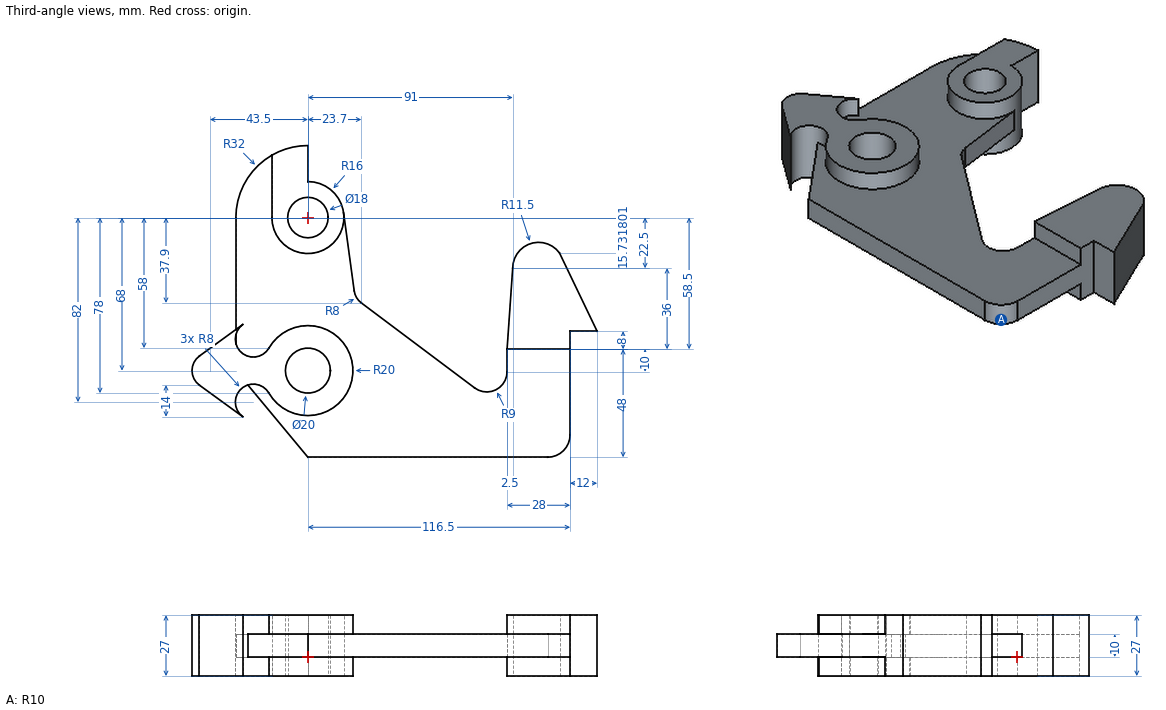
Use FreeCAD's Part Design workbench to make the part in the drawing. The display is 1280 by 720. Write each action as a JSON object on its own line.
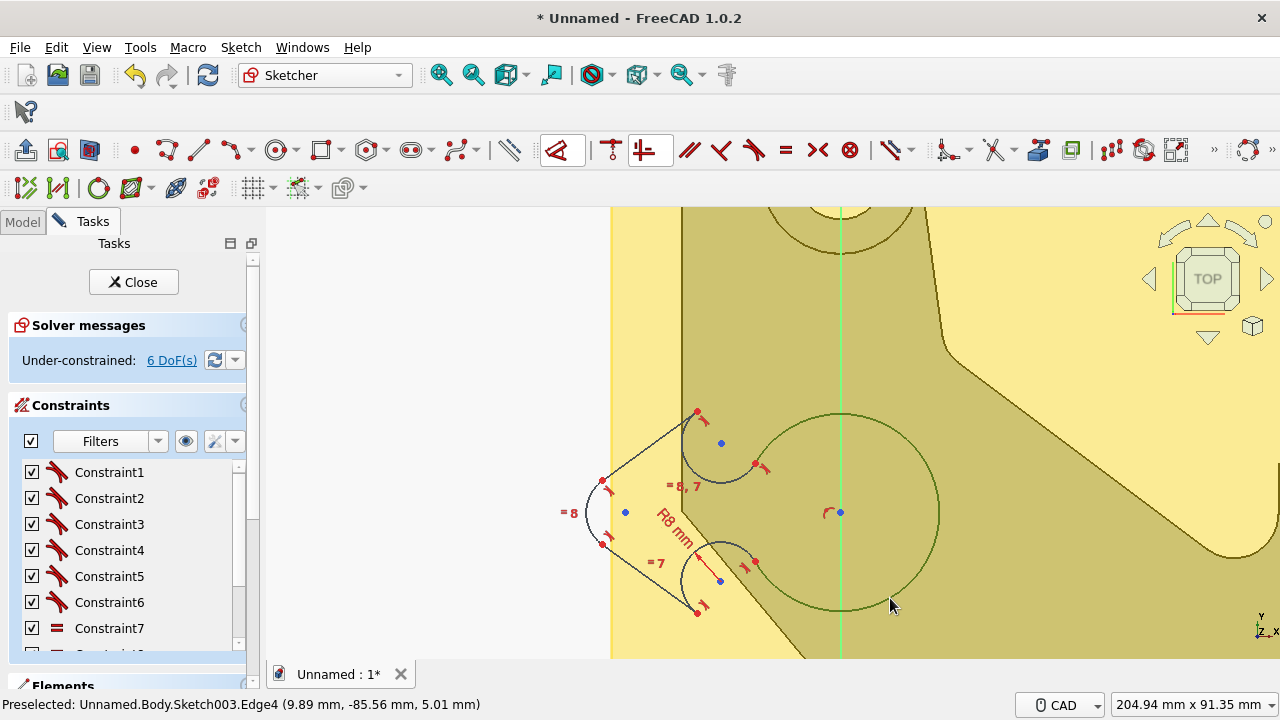
{"action": "key", "text": "k r"}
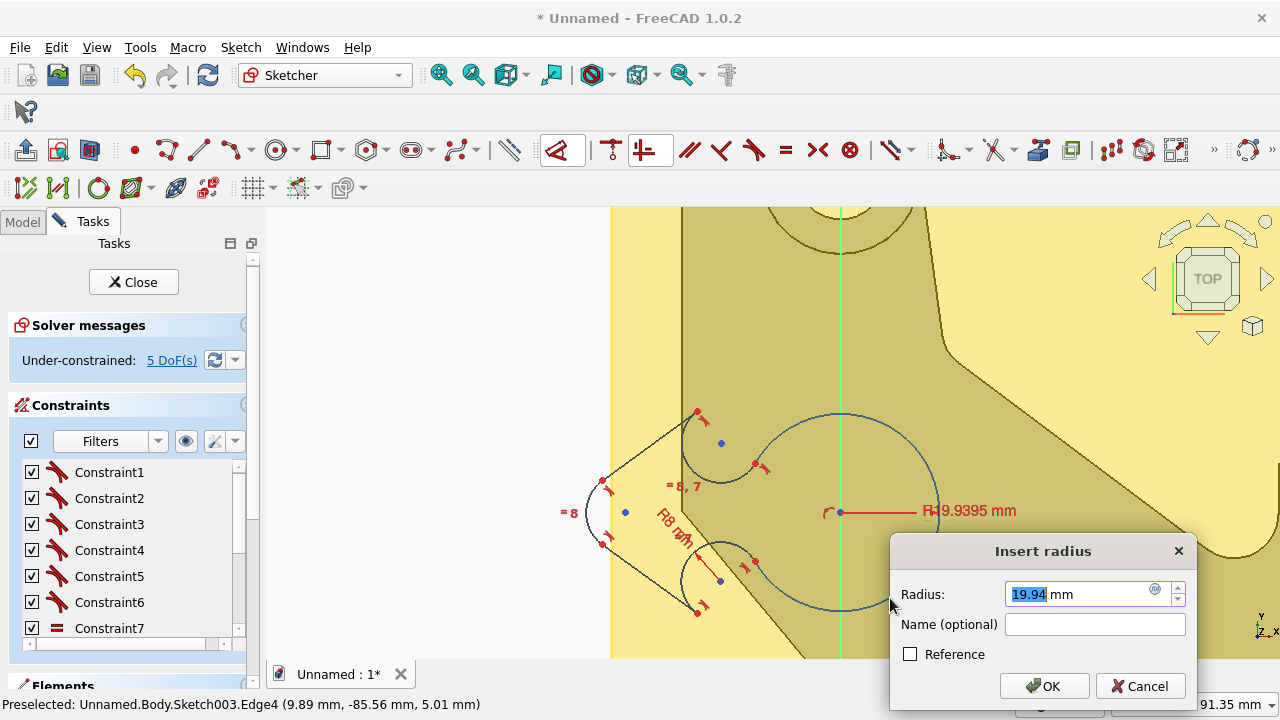
{"action": "type", "text": "20"}
{"action": "key", "text": "Return"}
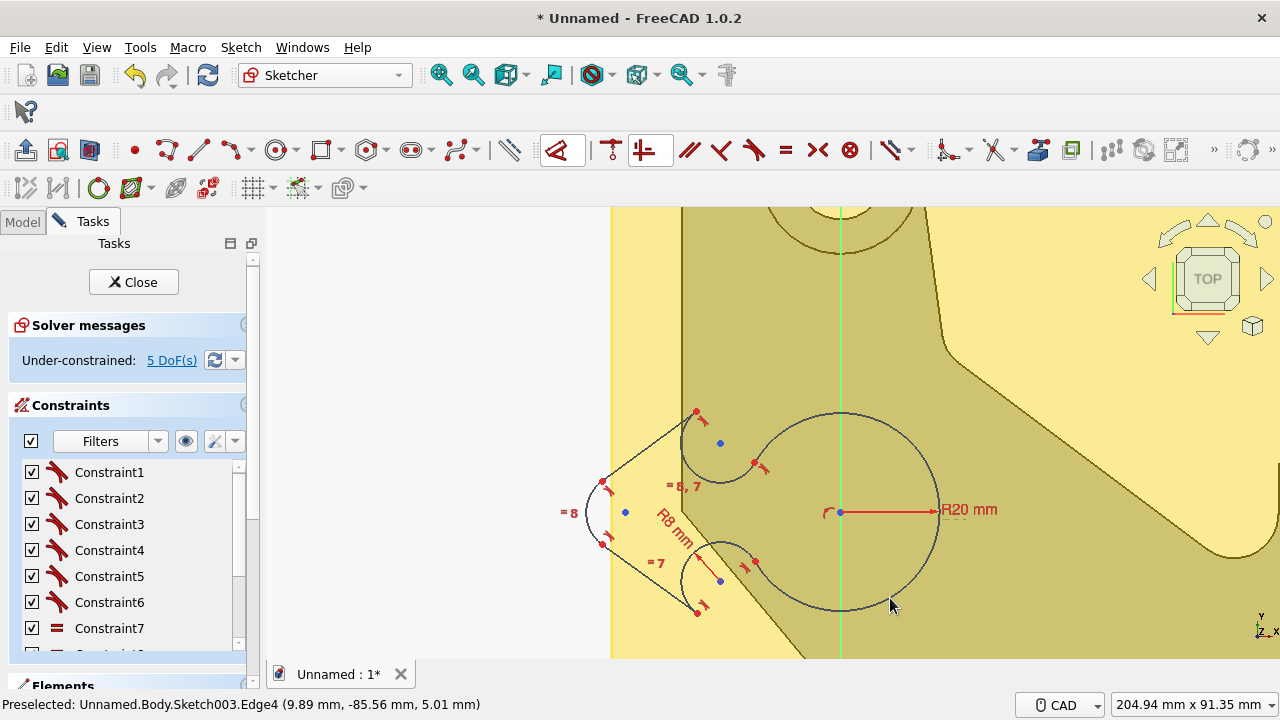
{"action": "left_click", "coordinate": [755, 562]}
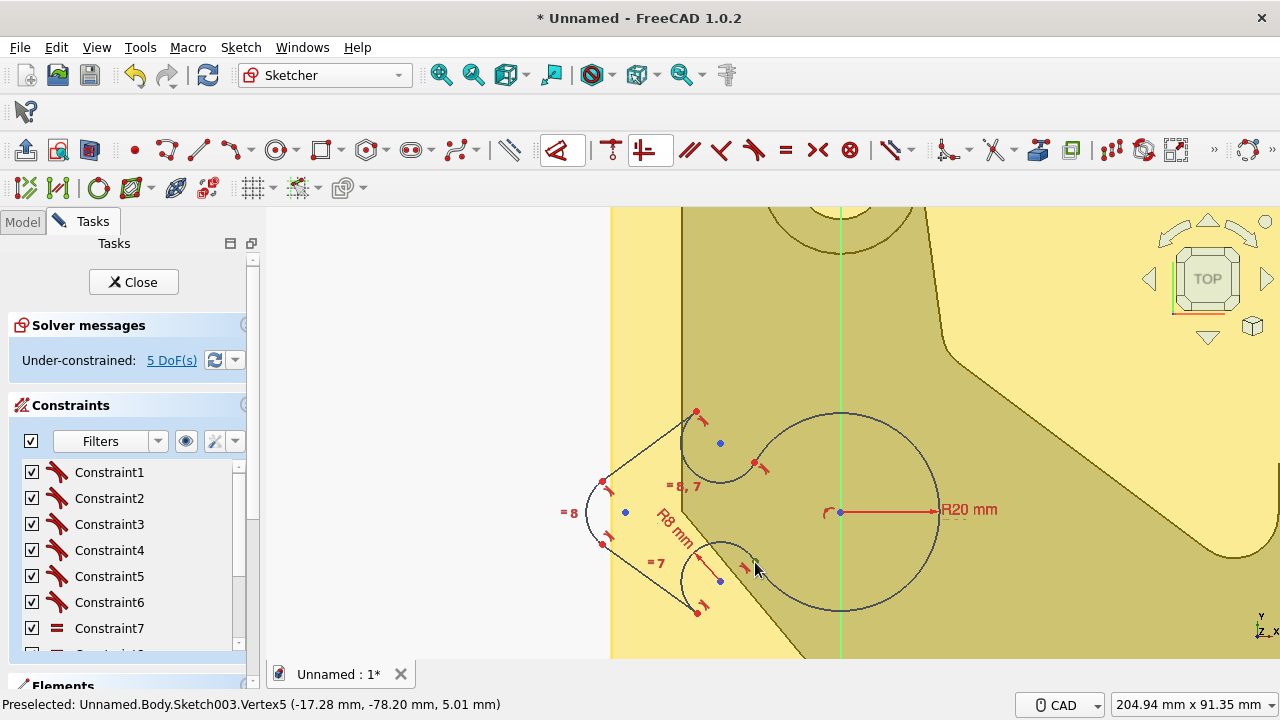
{"action": "left_click", "coordinate": [580, 150]}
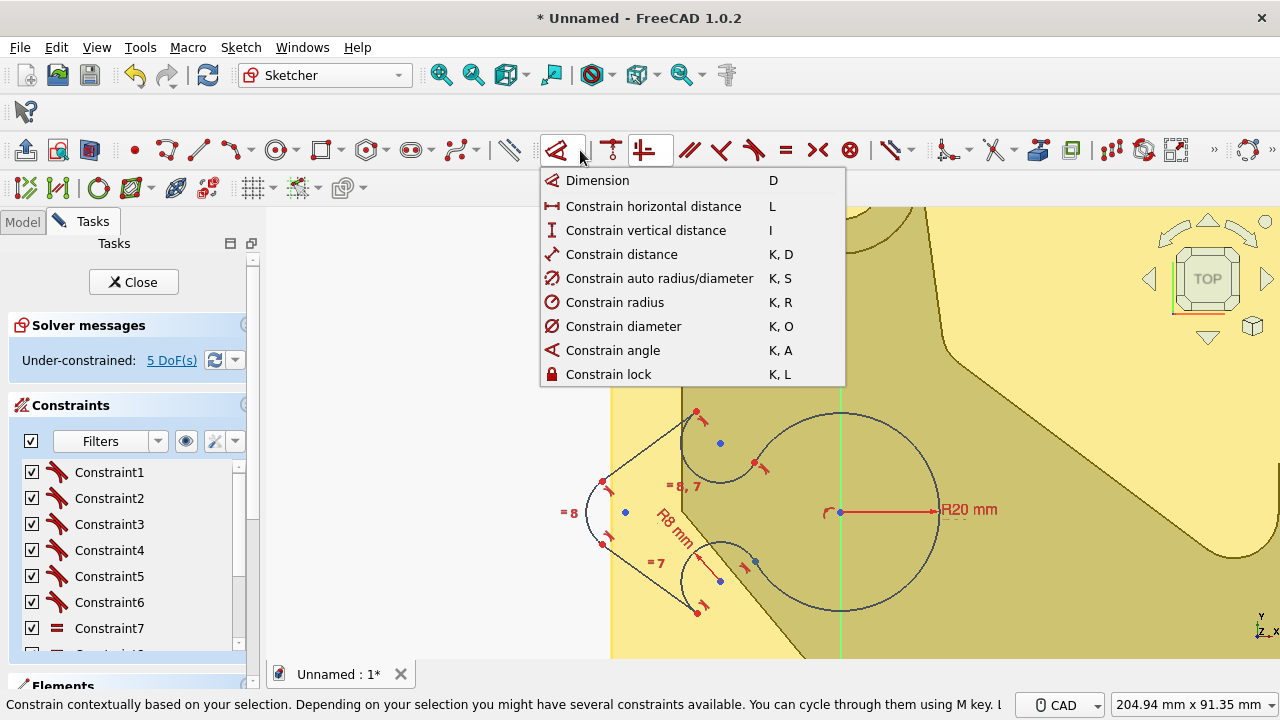
{"action": "left_click", "coordinate": [693, 230]}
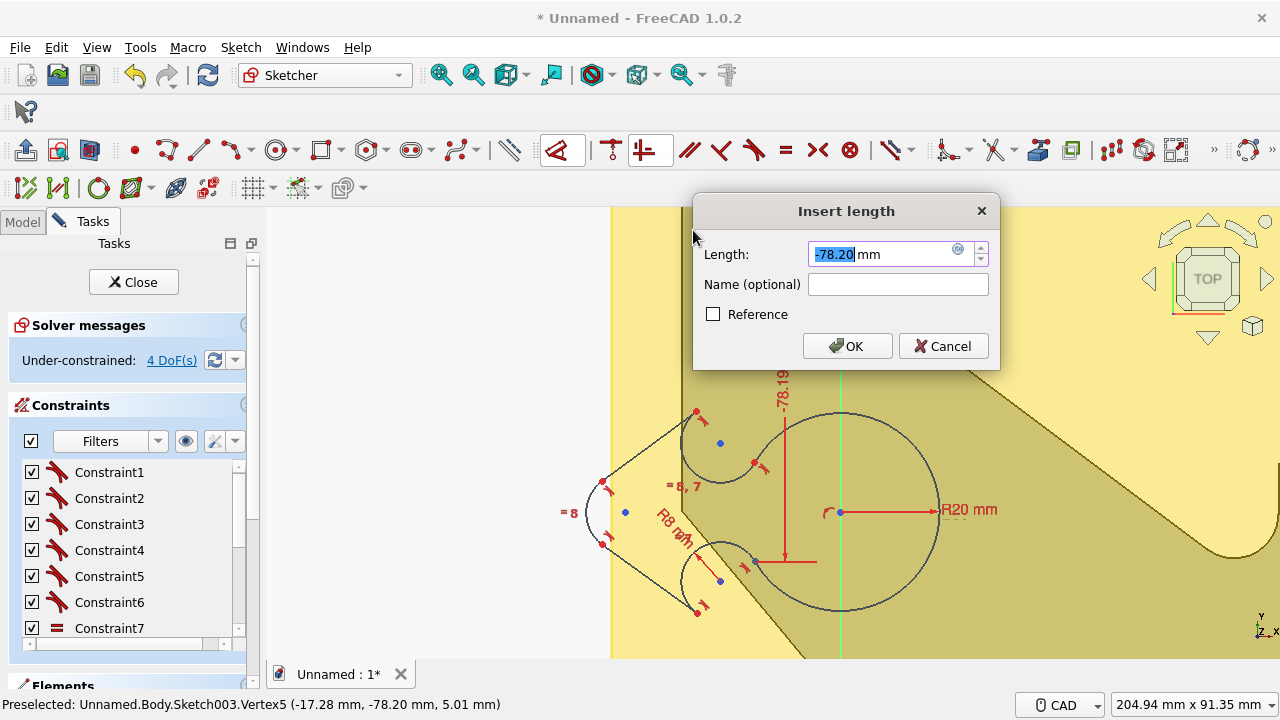
{"action": "type", "text": "-78"}
{"action": "key", "text": "Return"}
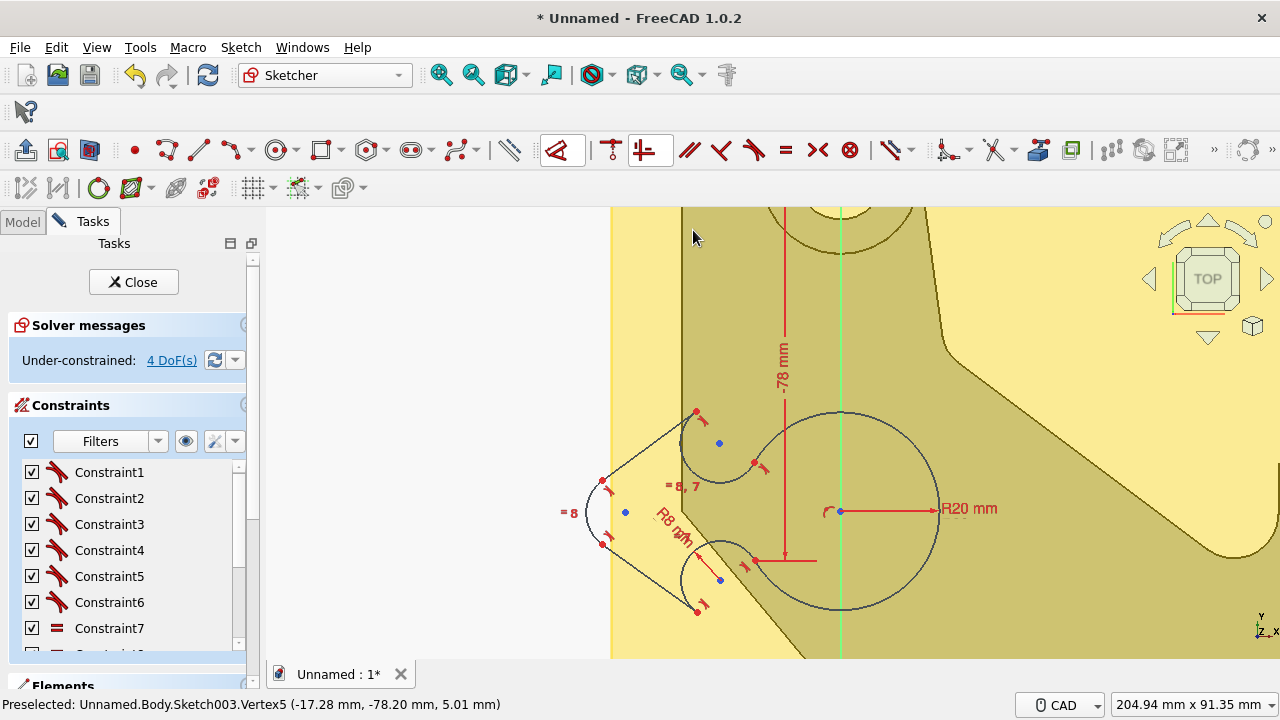
{"action": "left_click", "coordinate": [754, 463]}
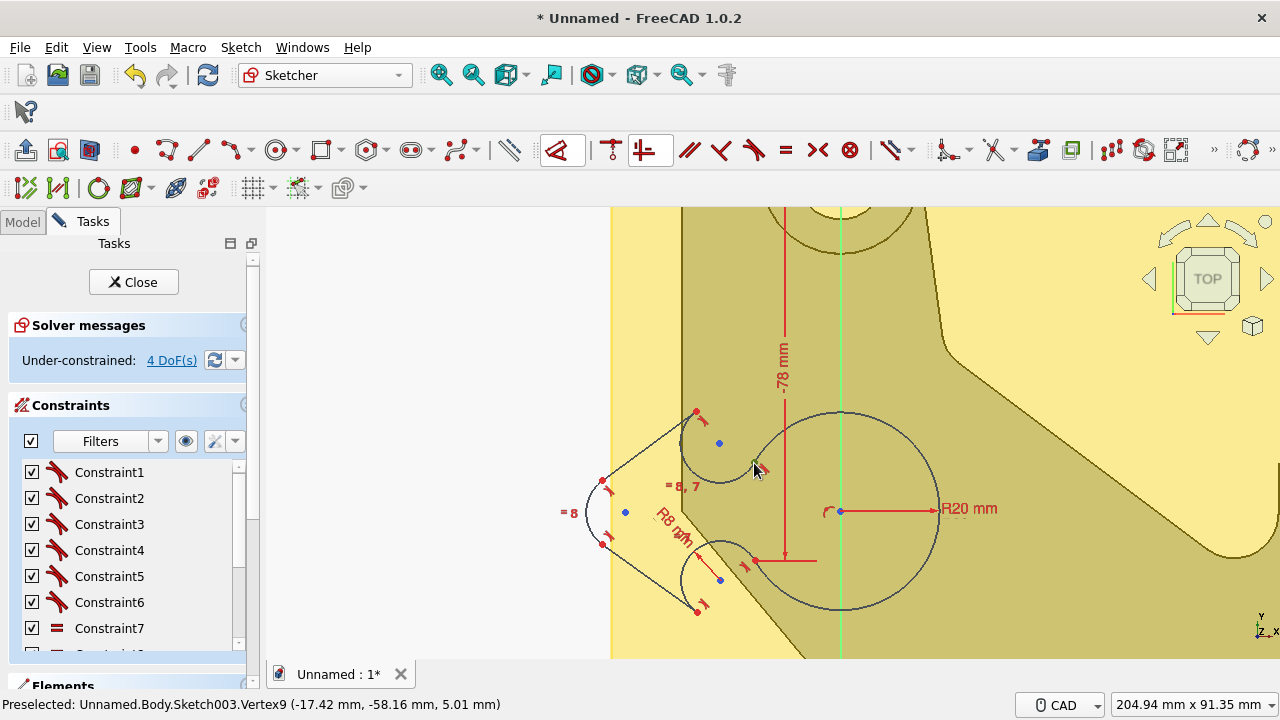
{"action": "key", "text": "i"}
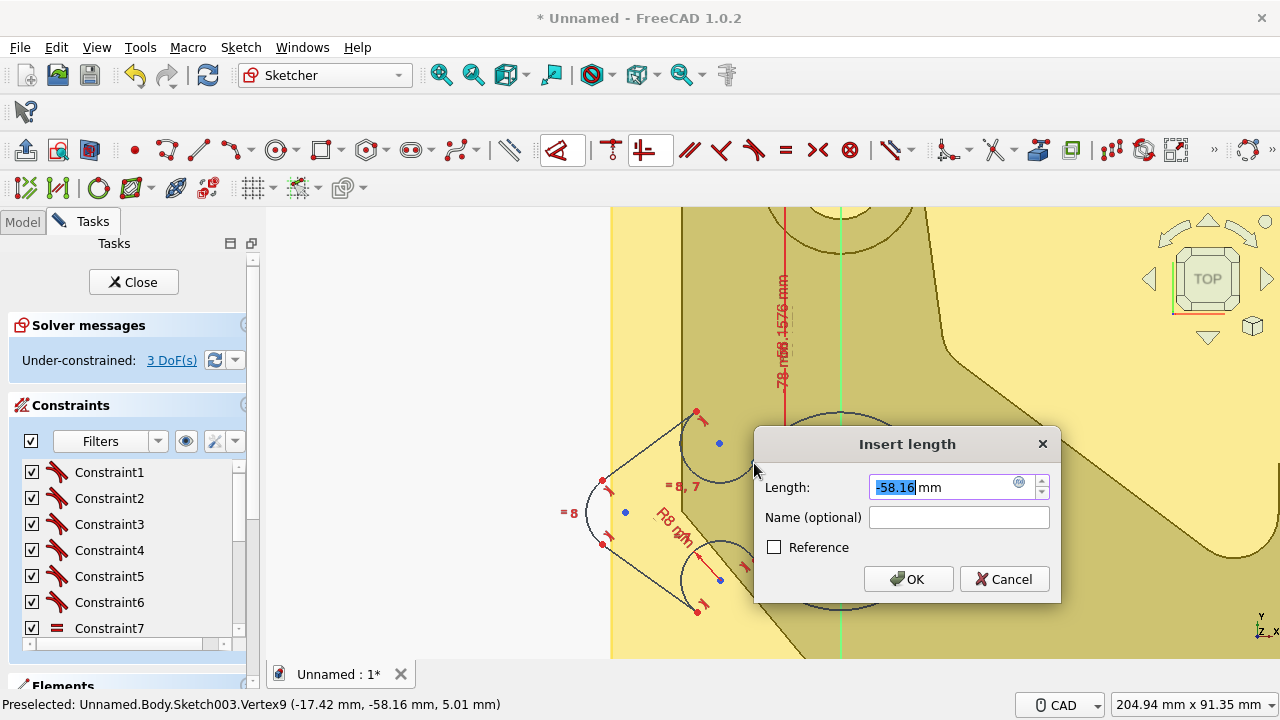
{"action": "type", "text": "-58"}
{"action": "key", "text": "Return"}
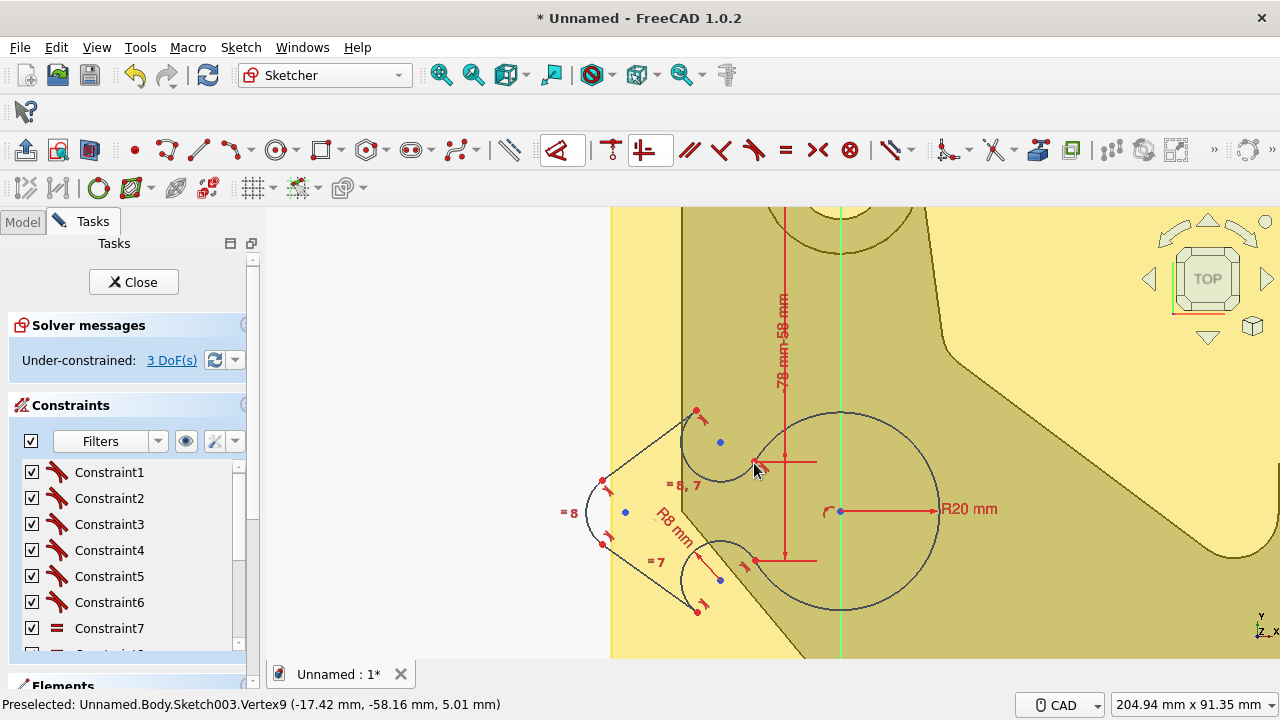
{"action": "left_click", "coordinate": [631, 565]}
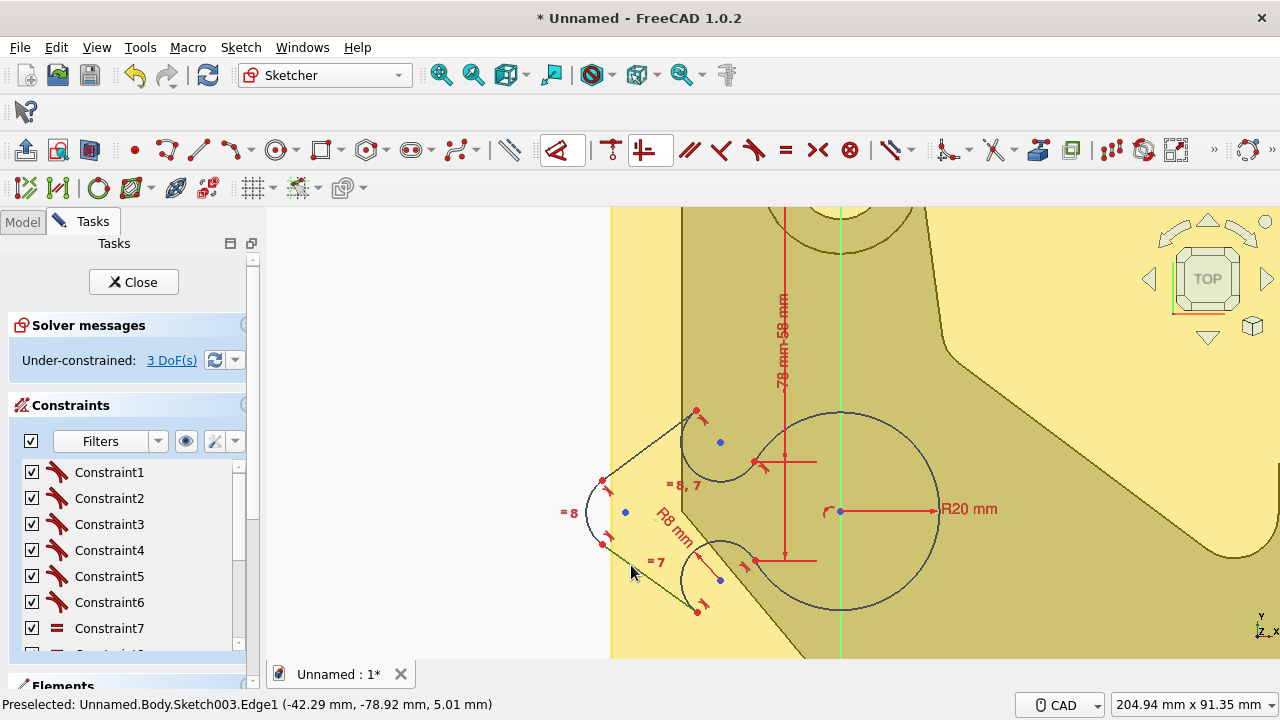
{"action": "key", "text": "i"}